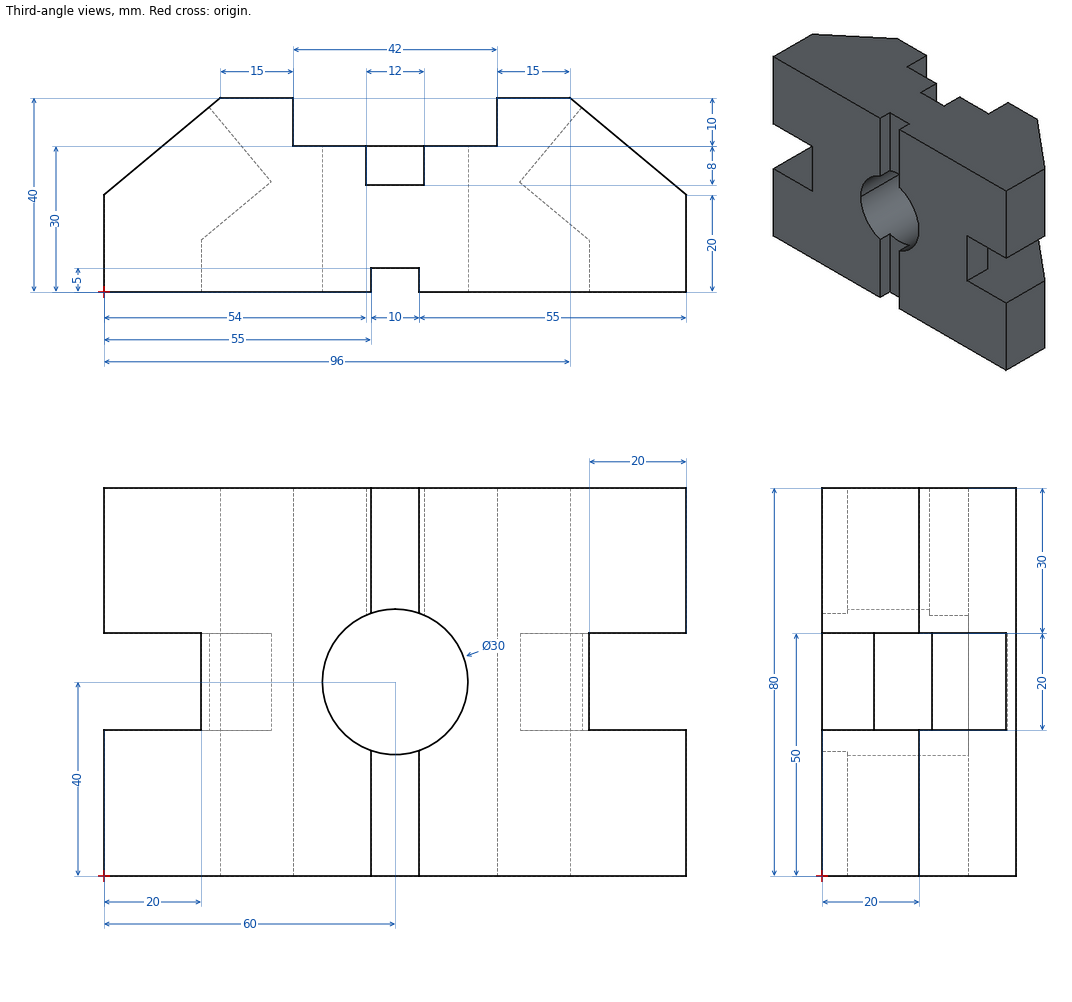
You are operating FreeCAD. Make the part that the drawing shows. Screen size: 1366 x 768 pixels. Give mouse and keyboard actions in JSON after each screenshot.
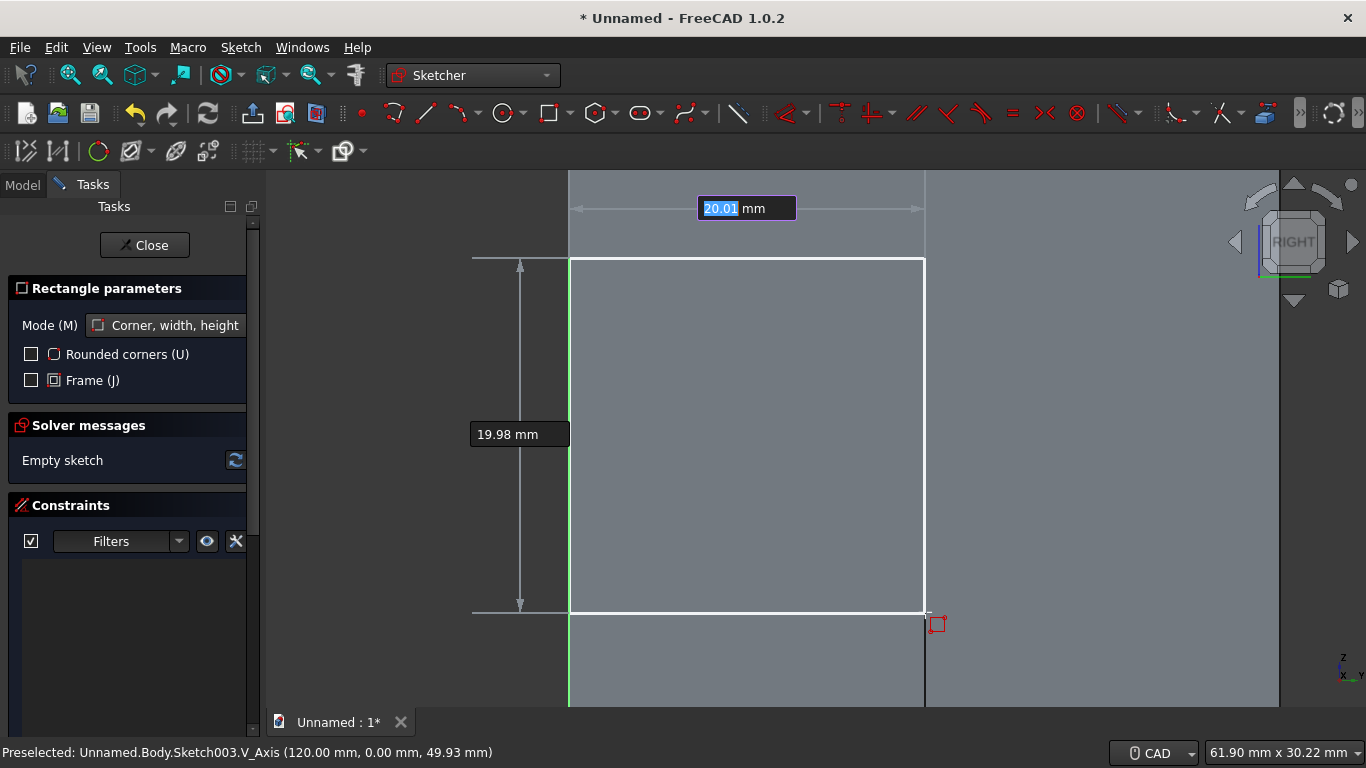
{"action": "type", "text": "20"}
{"action": "key", "text": "Tab"}
{"action": "type", "text": "20"}
{"action": "key", "text": "Return"}
{"action": "key", "text": "Escape"}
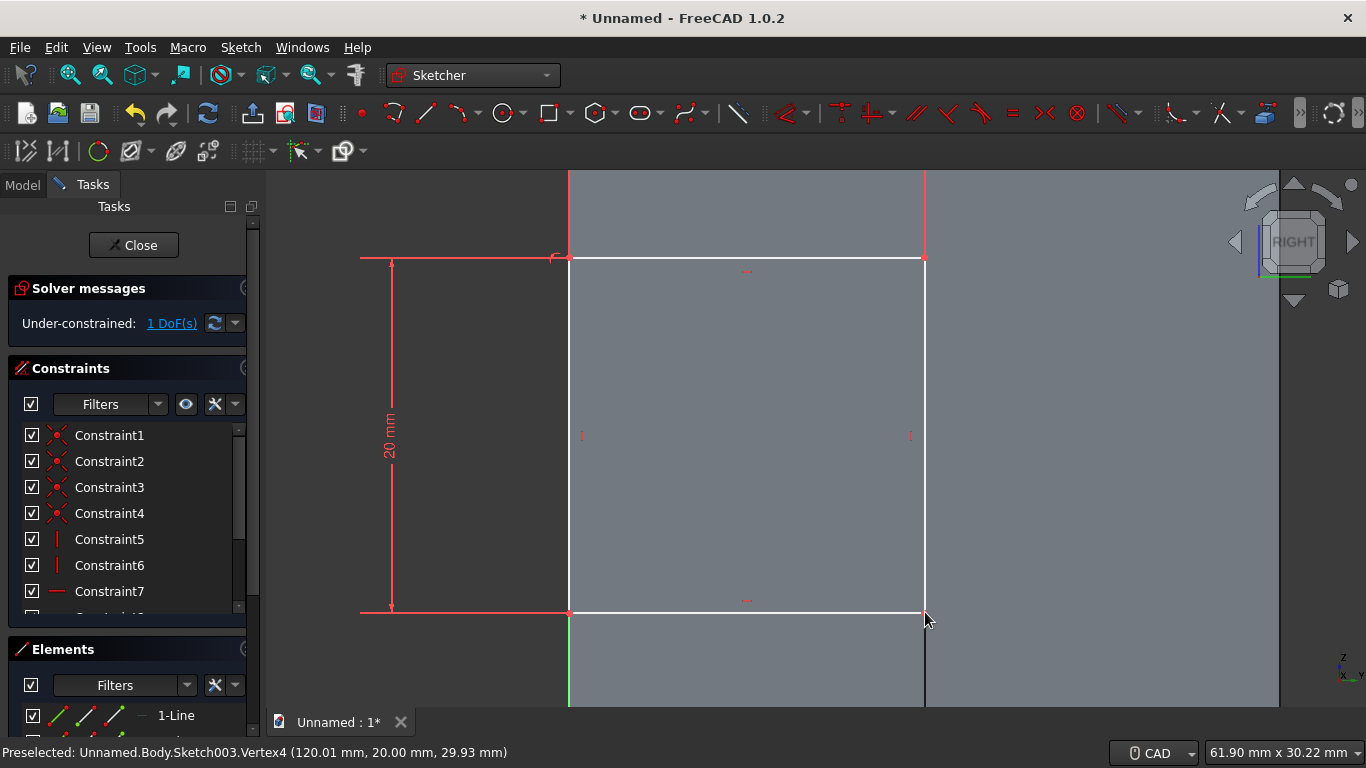
{"action": "key", "text": "d"}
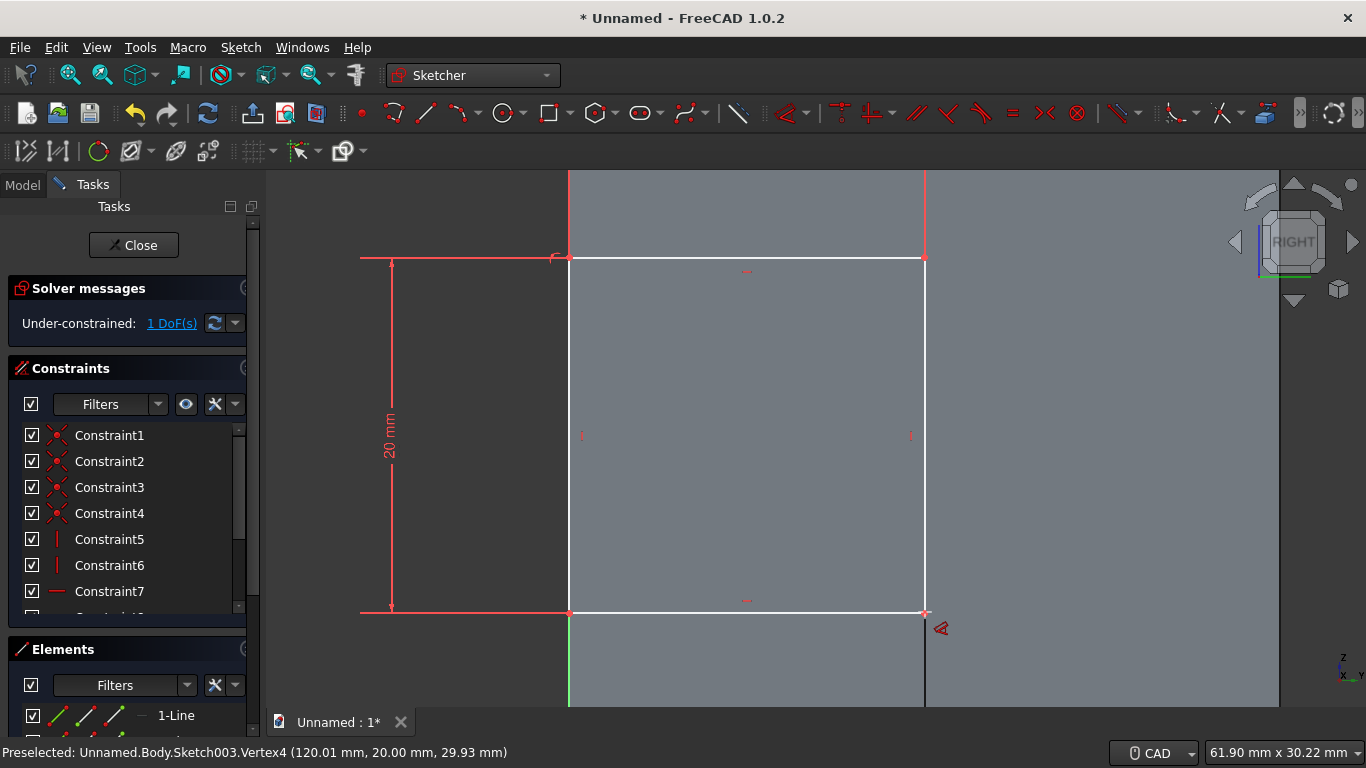
{"action": "left_click", "coordinate": [569, 258]}
{"action": "left_click", "coordinate": [535, 468]}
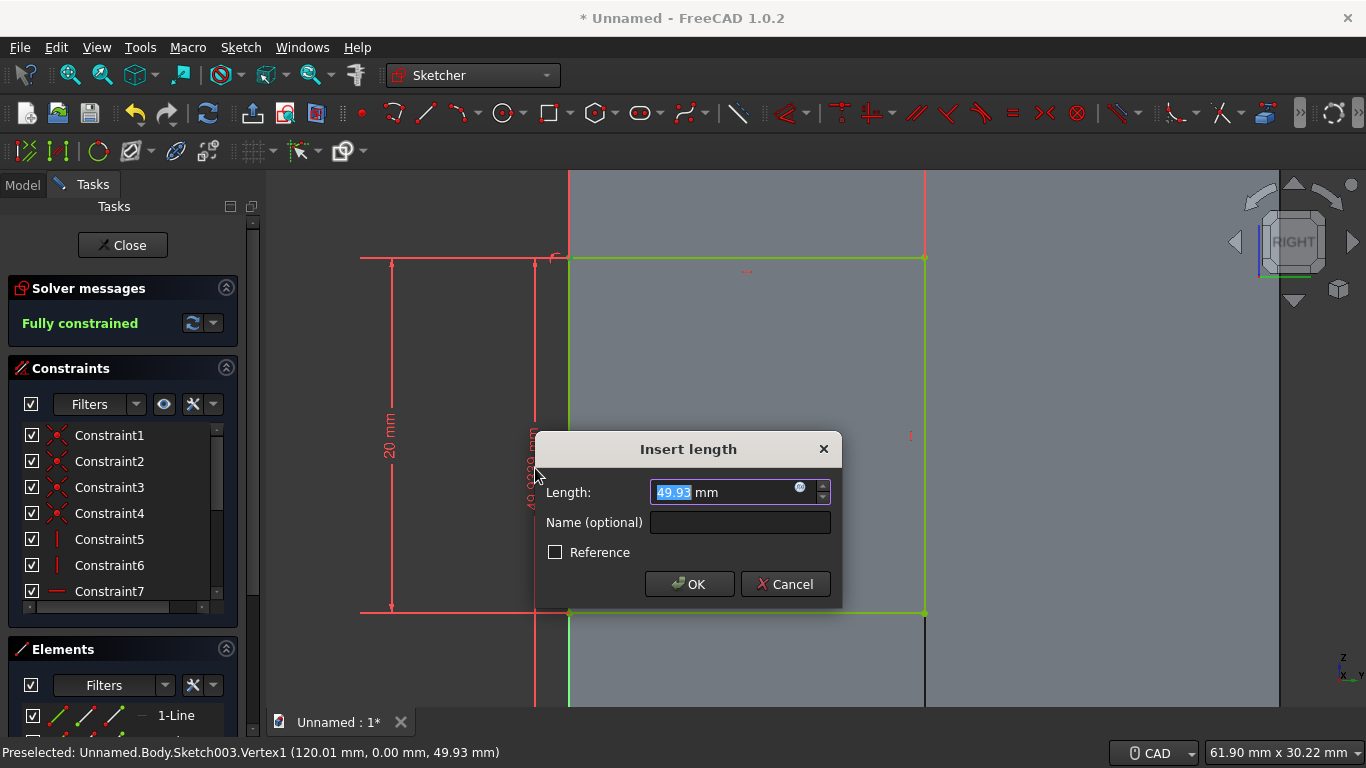
{"action": "type", "text": "50"}
{"action": "key", "text": "Return"}
{"action": "key", "text": "Escape"}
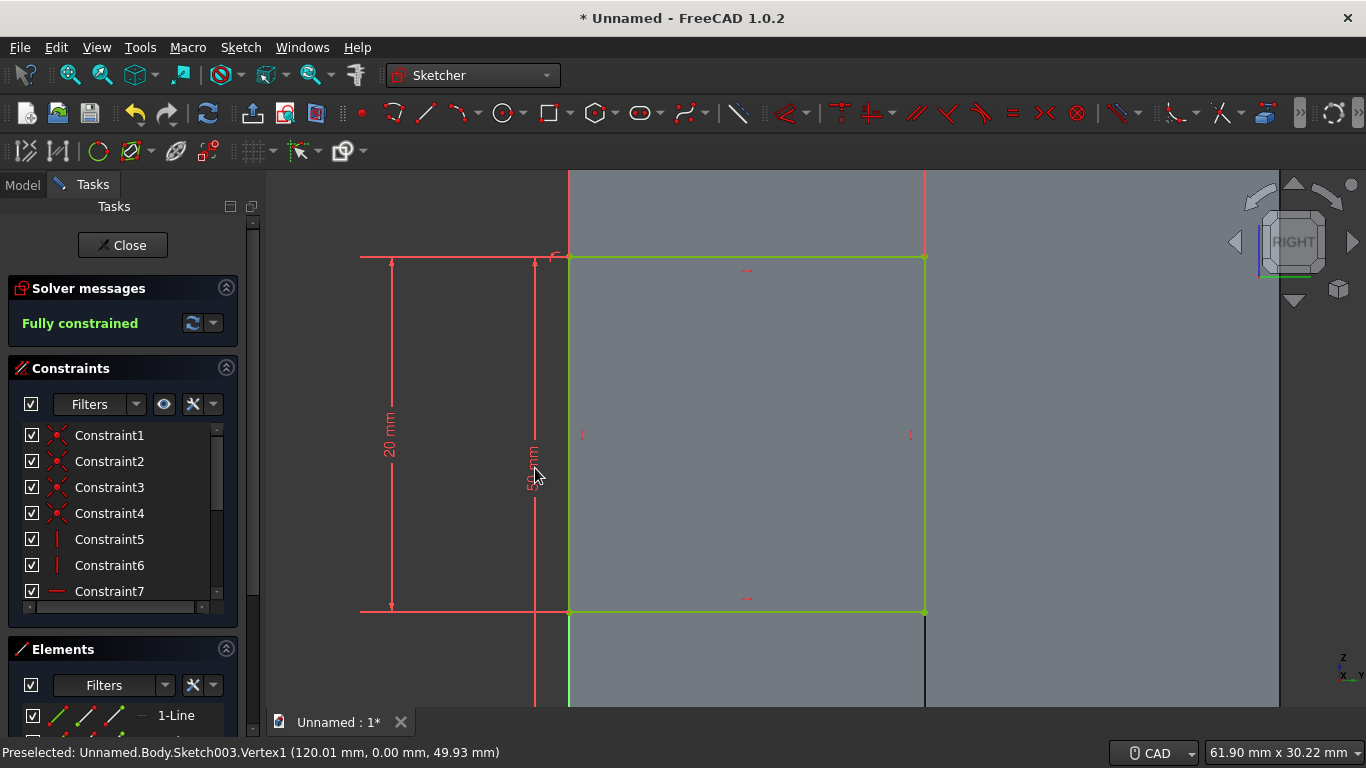
{"action": "left_click", "coordinate": [123, 245]}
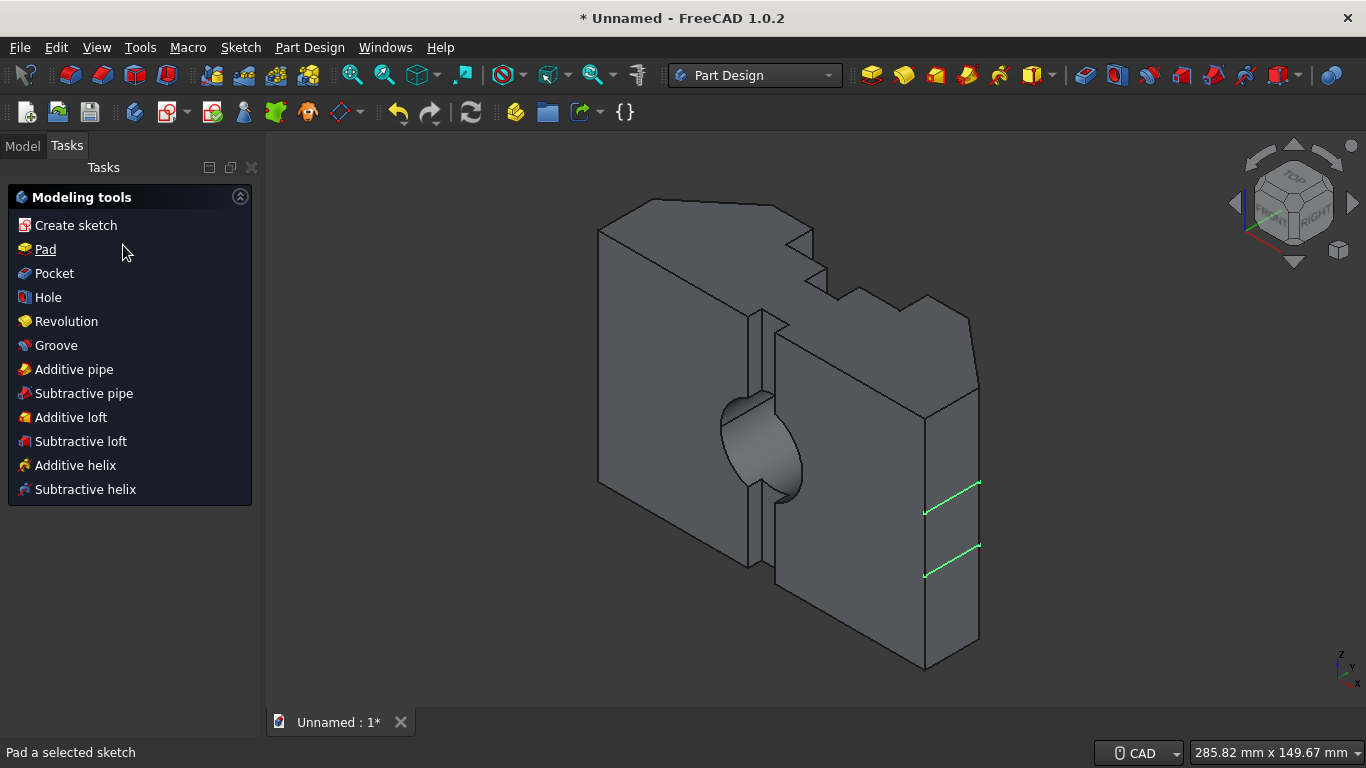
{"action": "left_click", "coordinate": [1086, 76]}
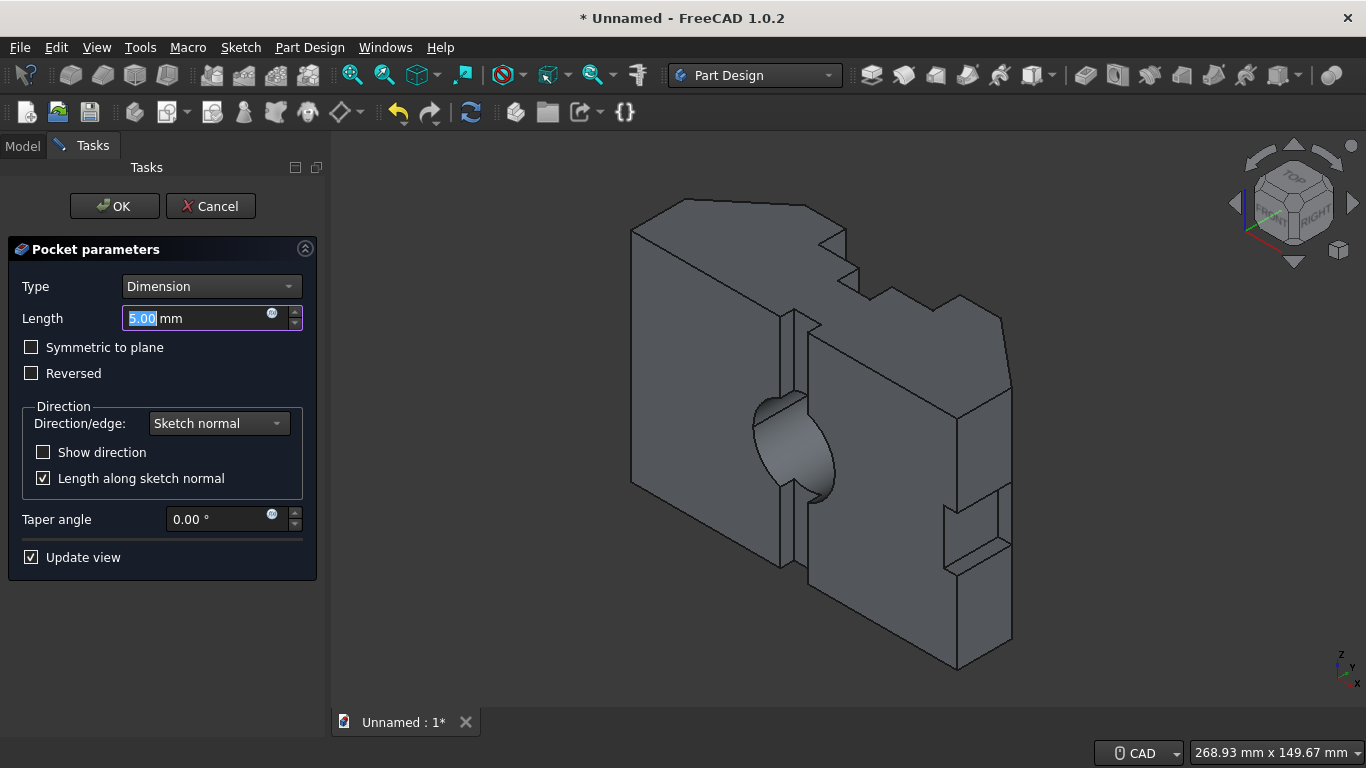
{"action": "type", "text": "20"}
{"action": "key", "text": "Tab"}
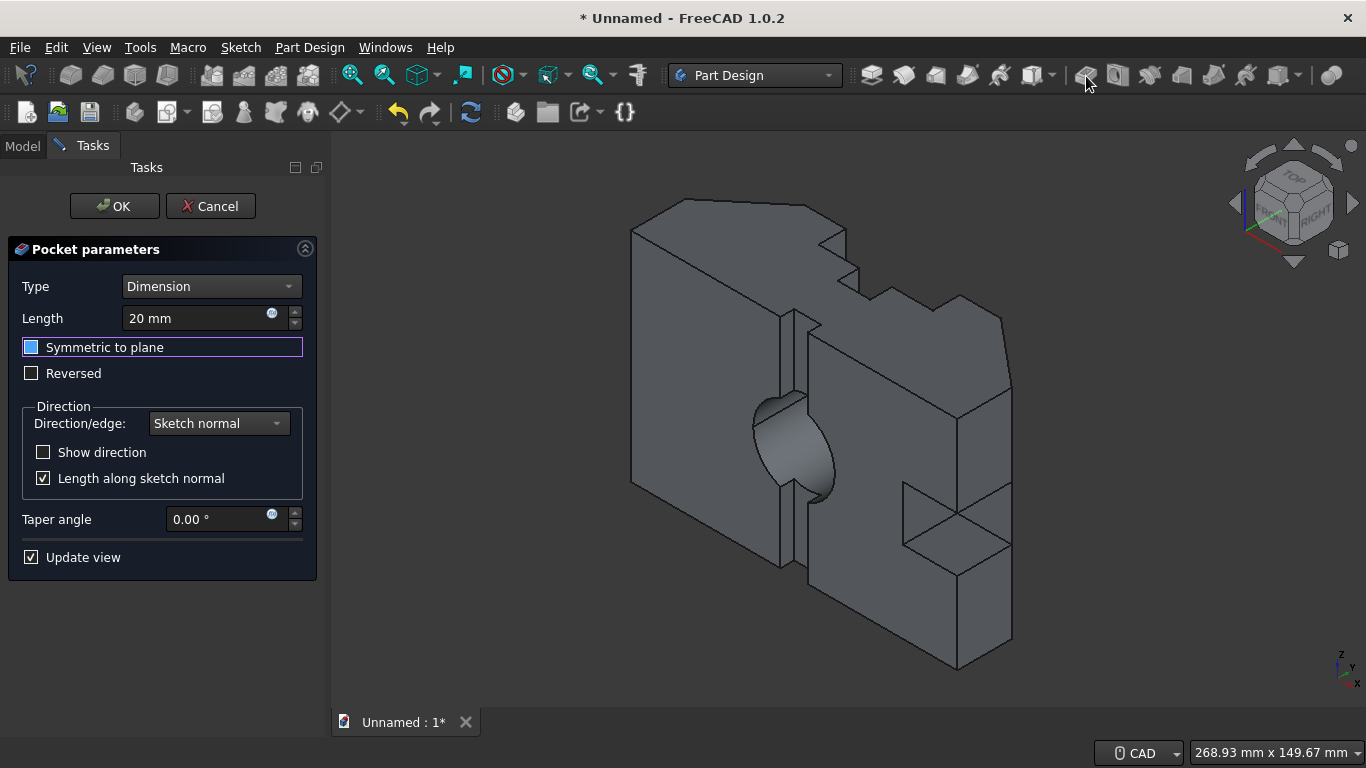
{"action": "left_click", "coordinate": [115, 206]}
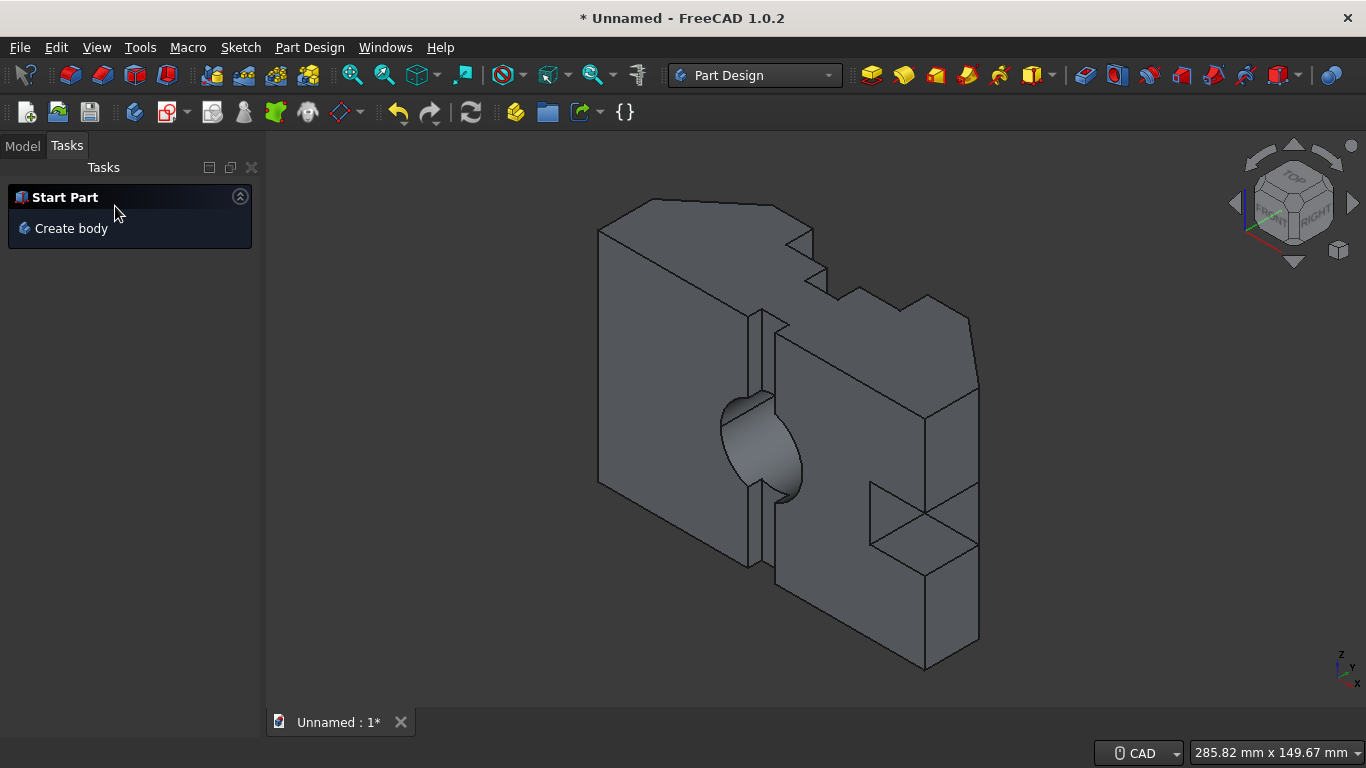
{"action": "key", "text": "4"}